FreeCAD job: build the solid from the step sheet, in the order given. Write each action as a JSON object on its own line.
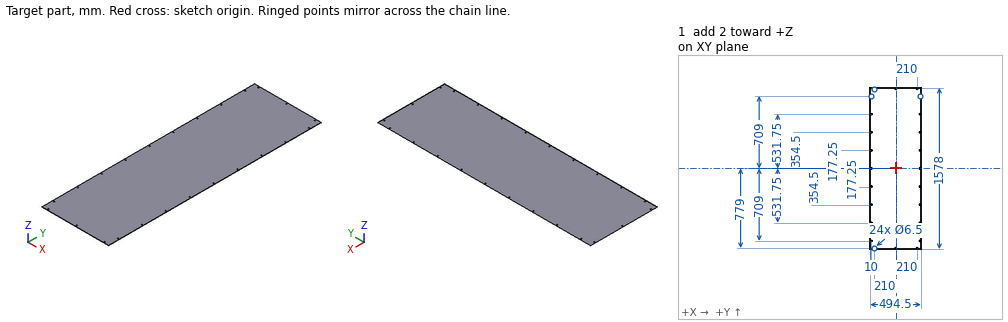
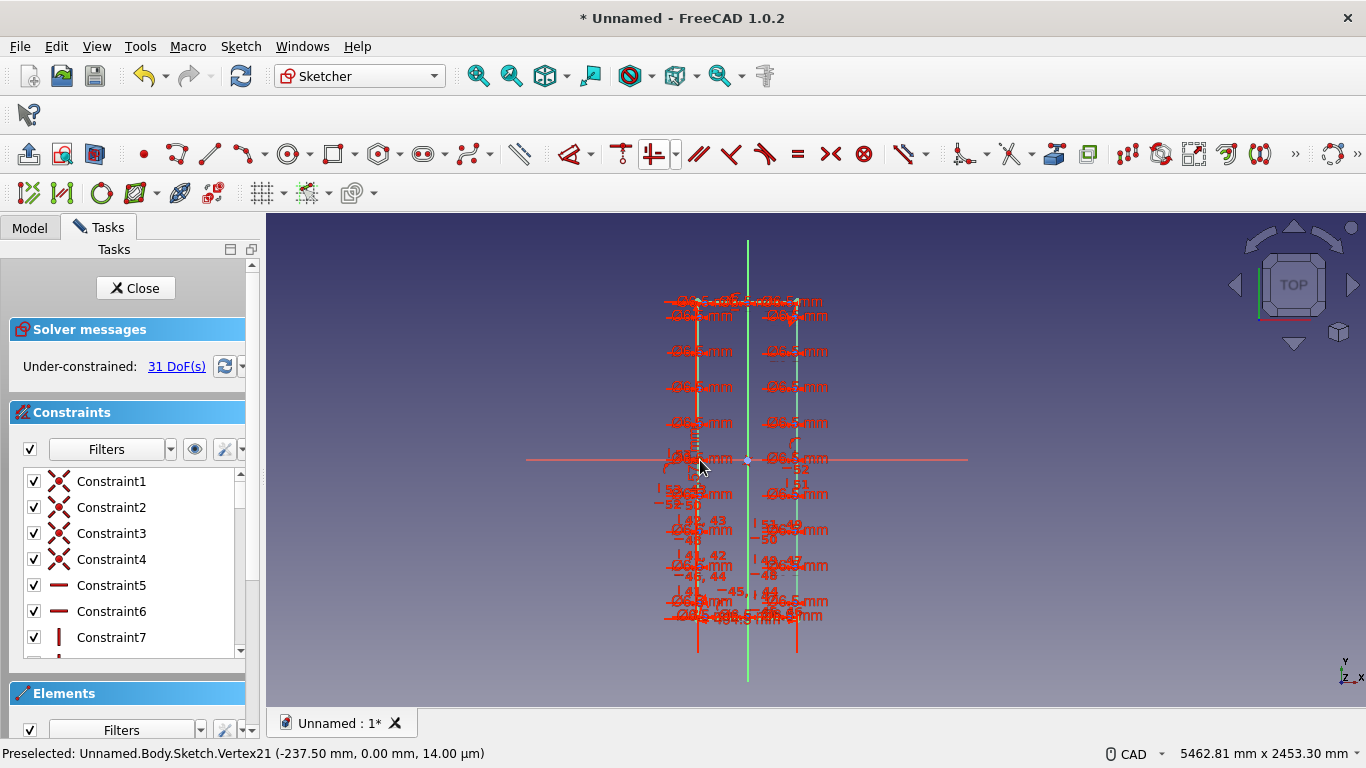
{"action": "left_click", "coordinate": [700, 425]}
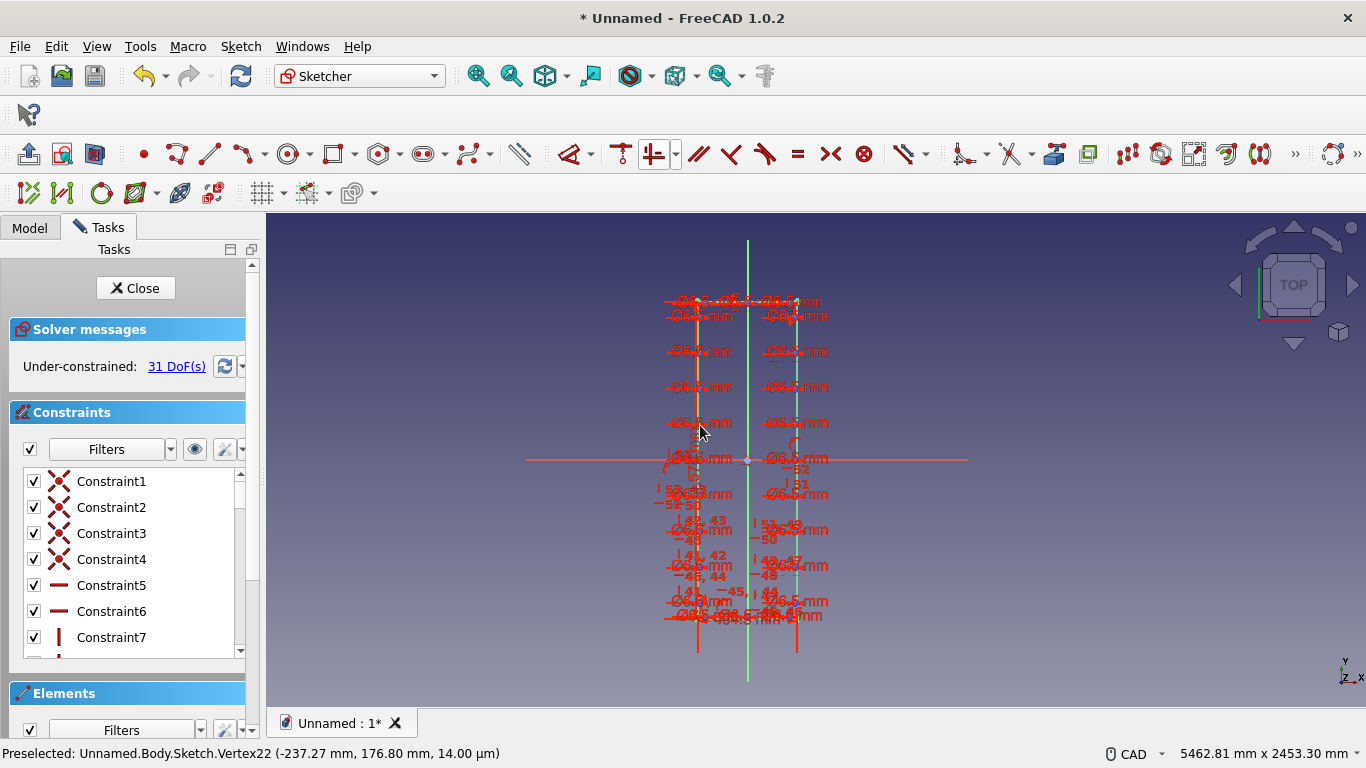
{"action": "key", "text": "v"}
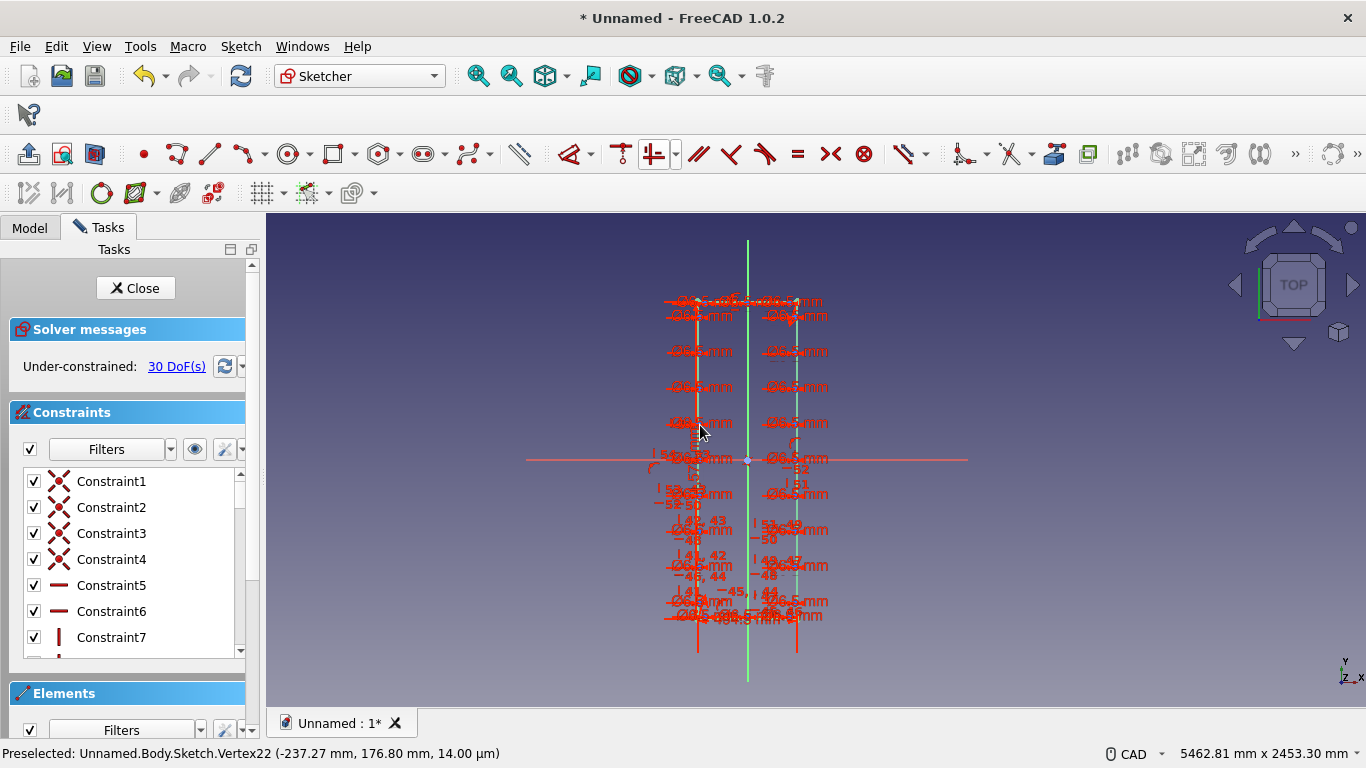
{"action": "left_click", "coordinate": [700, 425]}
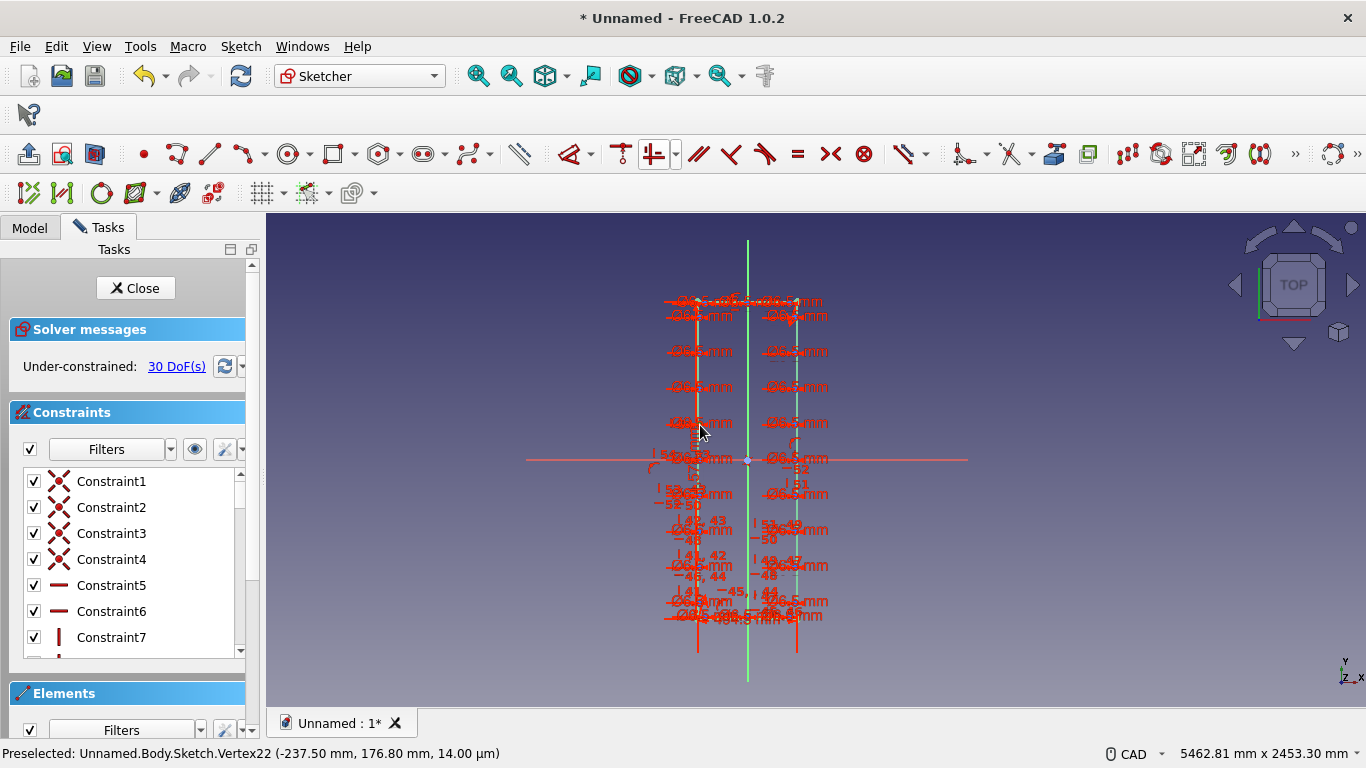
{"action": "left_click", "coordinate": [700, 389]}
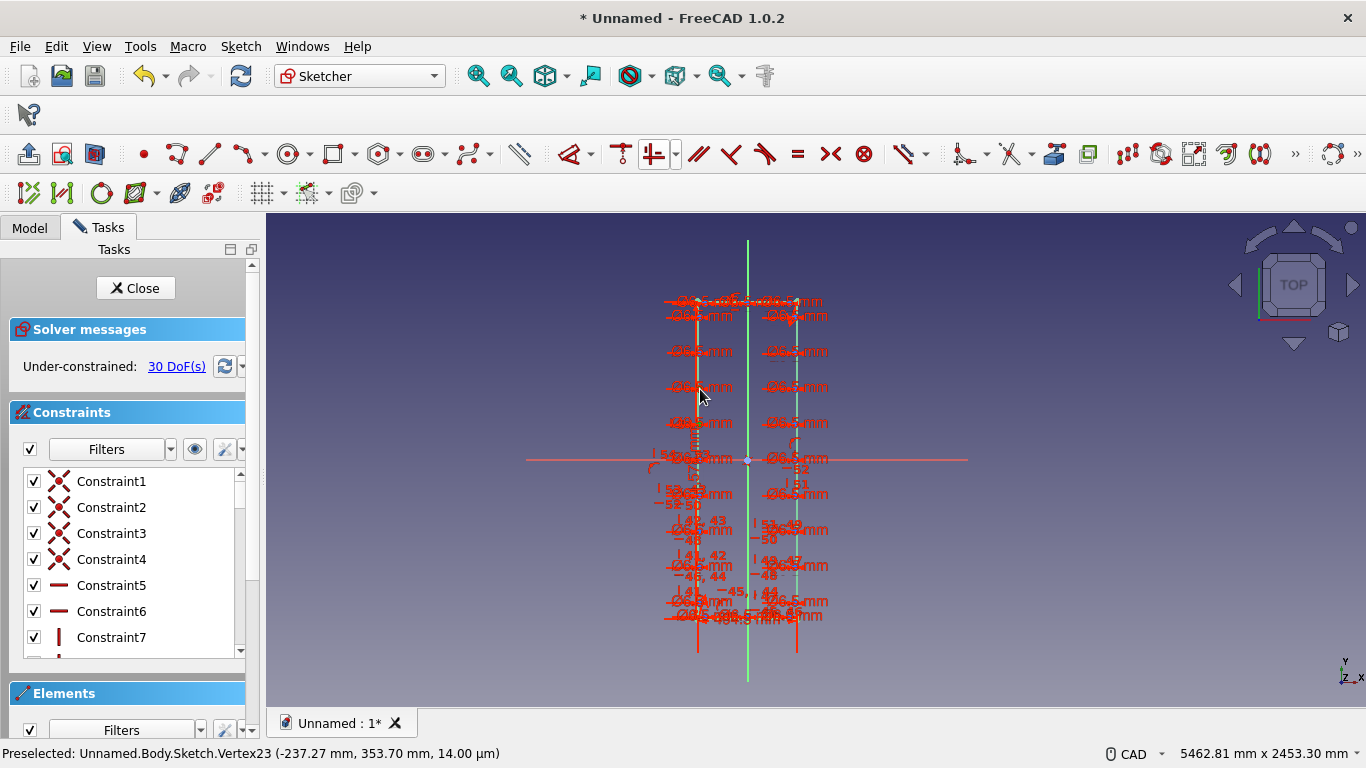
{"action": "key", "text": "v"}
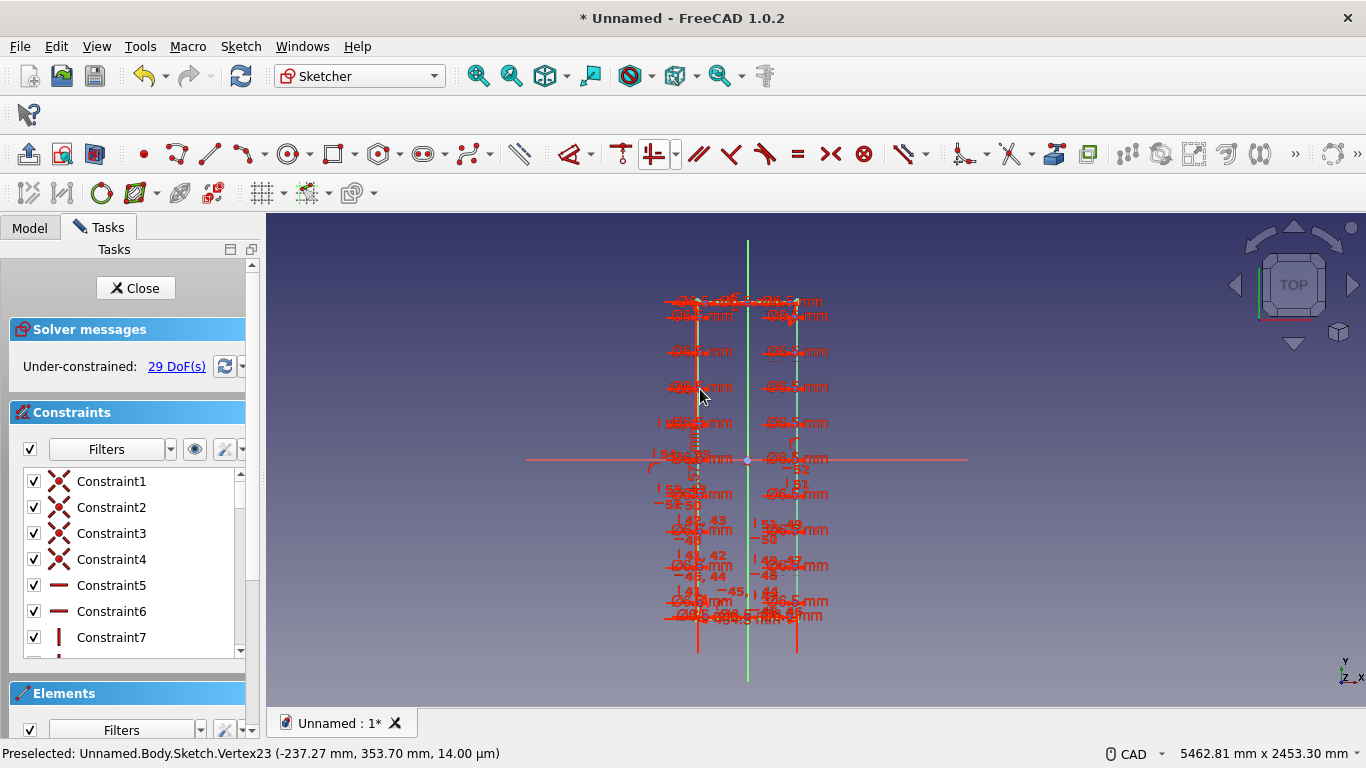
{"action": "left_click", "coordinate": [700, 389]}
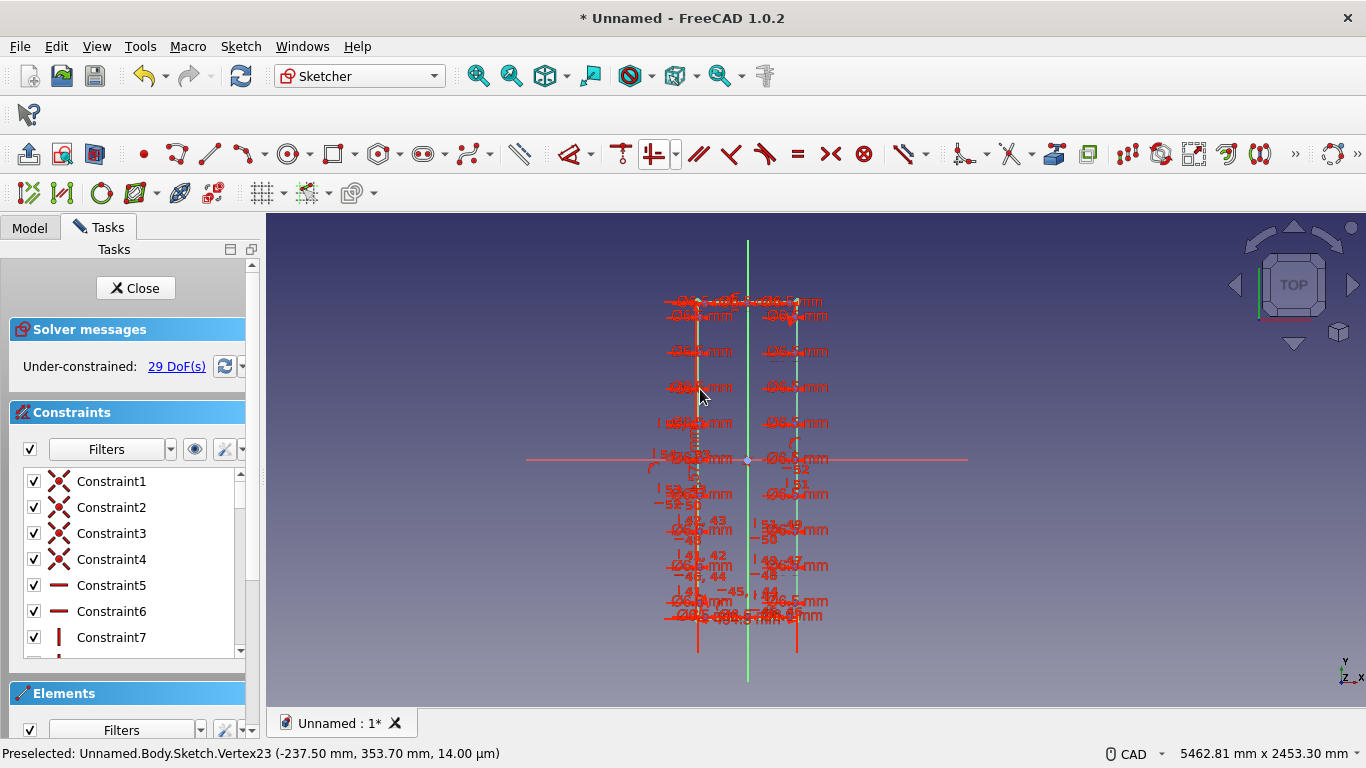
{"action": "left_click", "coordinate": [700, 353]}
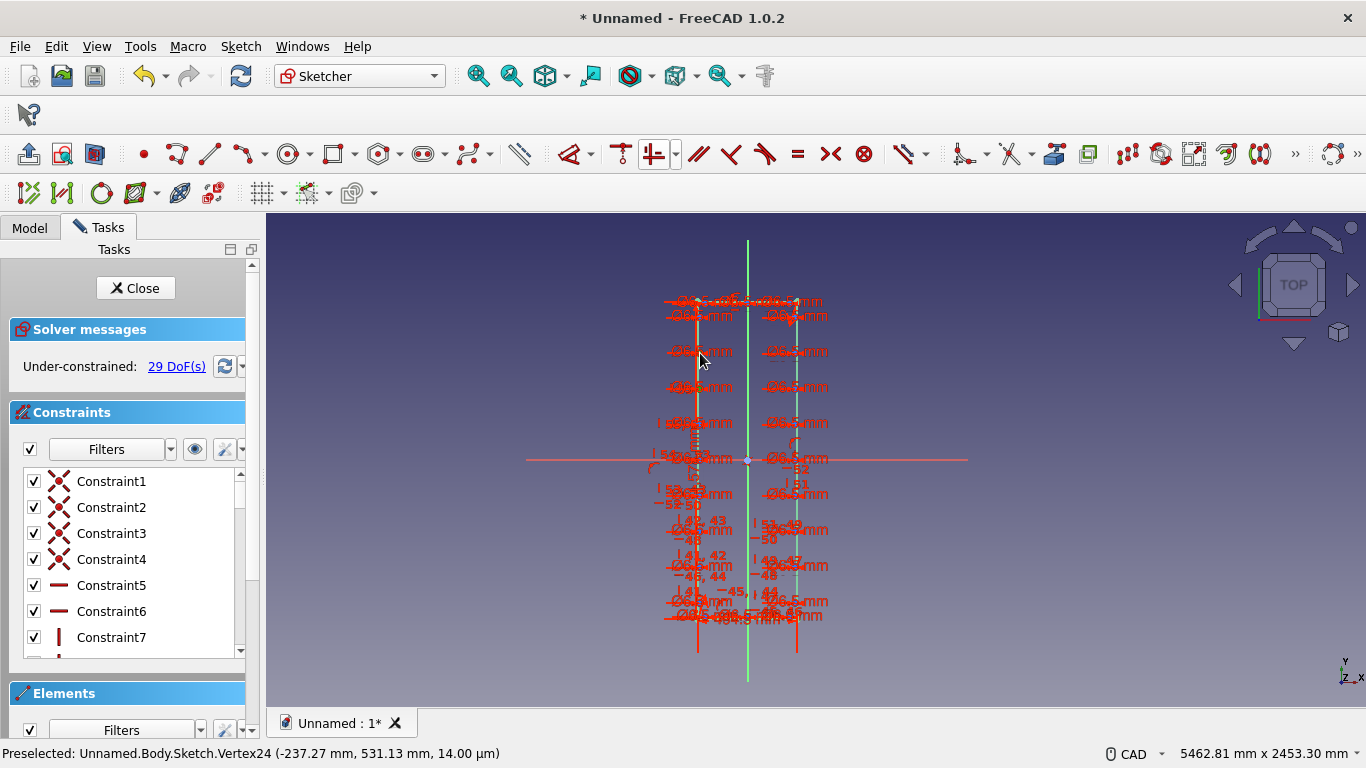
{"action": "left_click", "coordinate": [676, 154]}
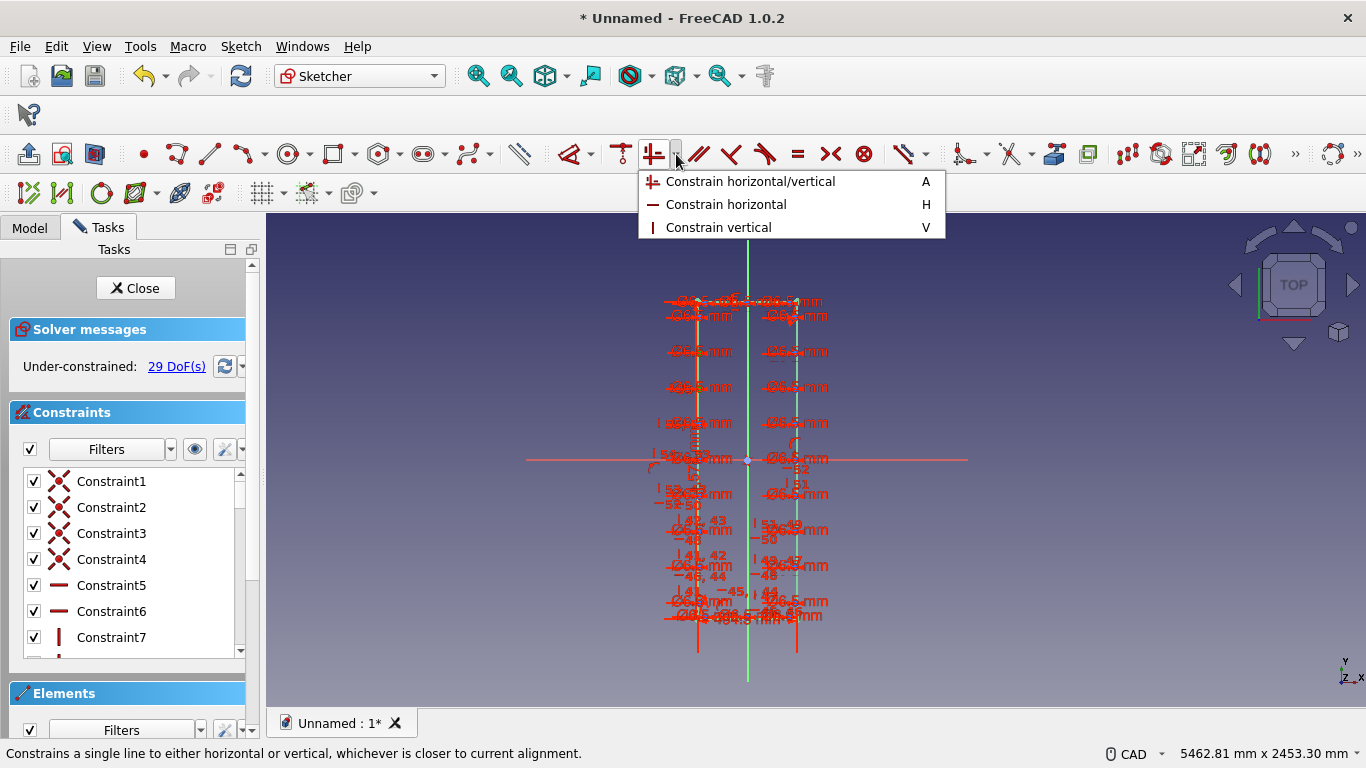
{"action": "left_click", "coordinate": [792, 228]}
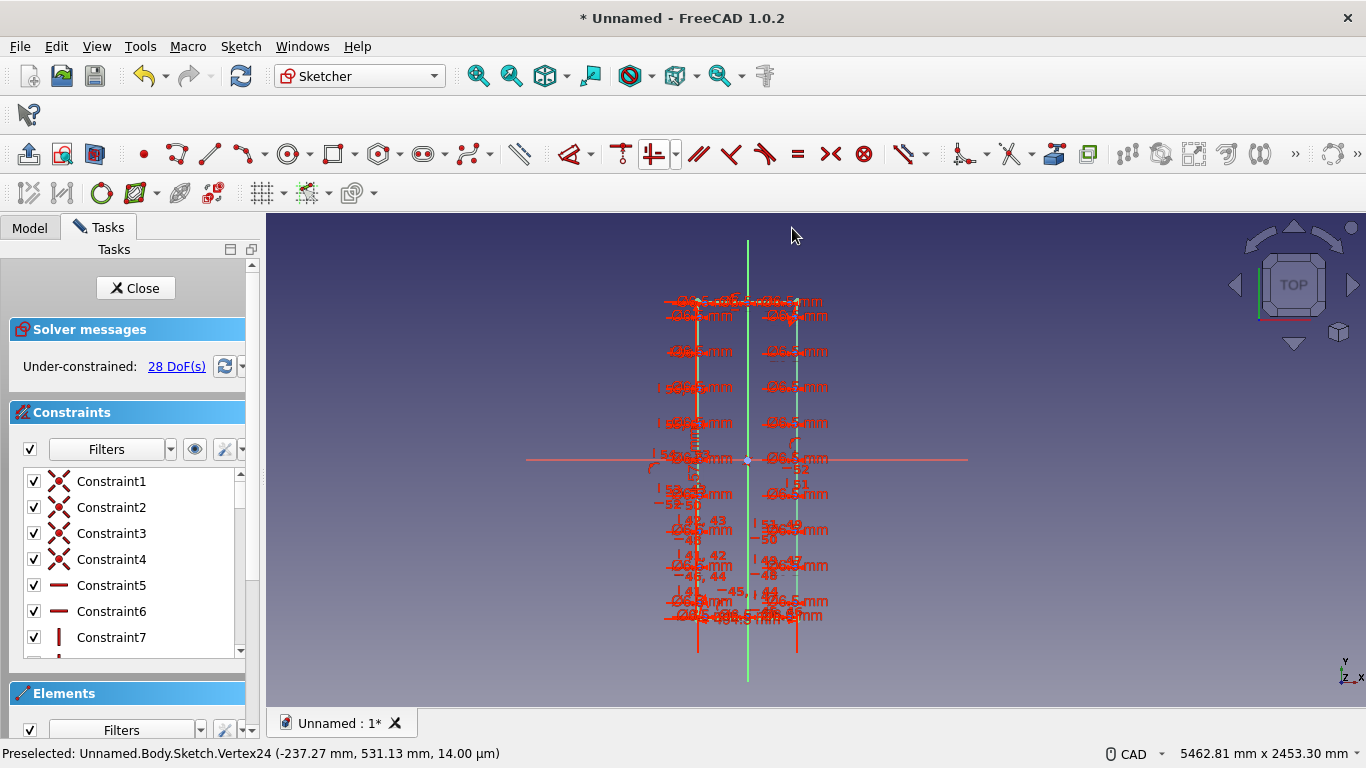
{"action": "left_click", "coordinate": [700, 353]}